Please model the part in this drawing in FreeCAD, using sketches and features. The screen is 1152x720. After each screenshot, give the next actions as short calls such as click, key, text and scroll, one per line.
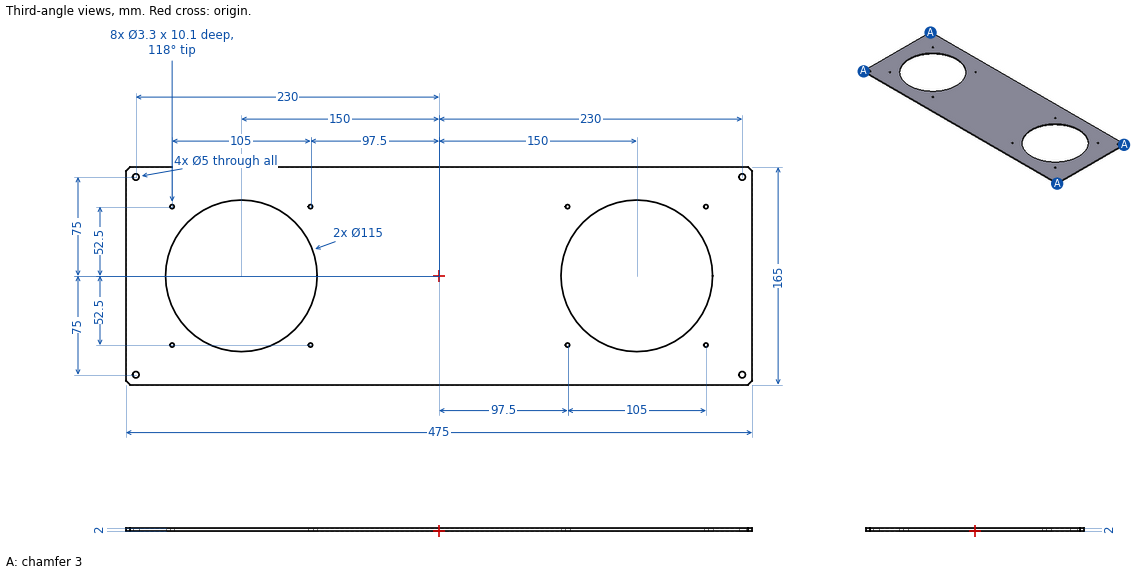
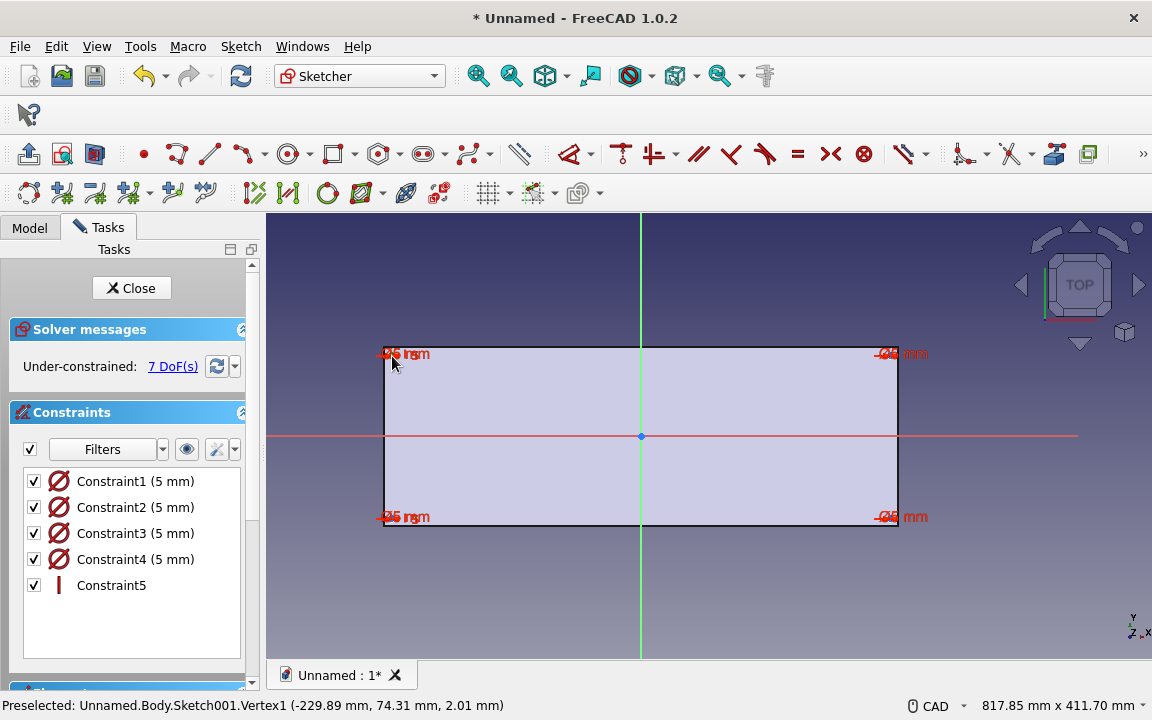
click(890, 356)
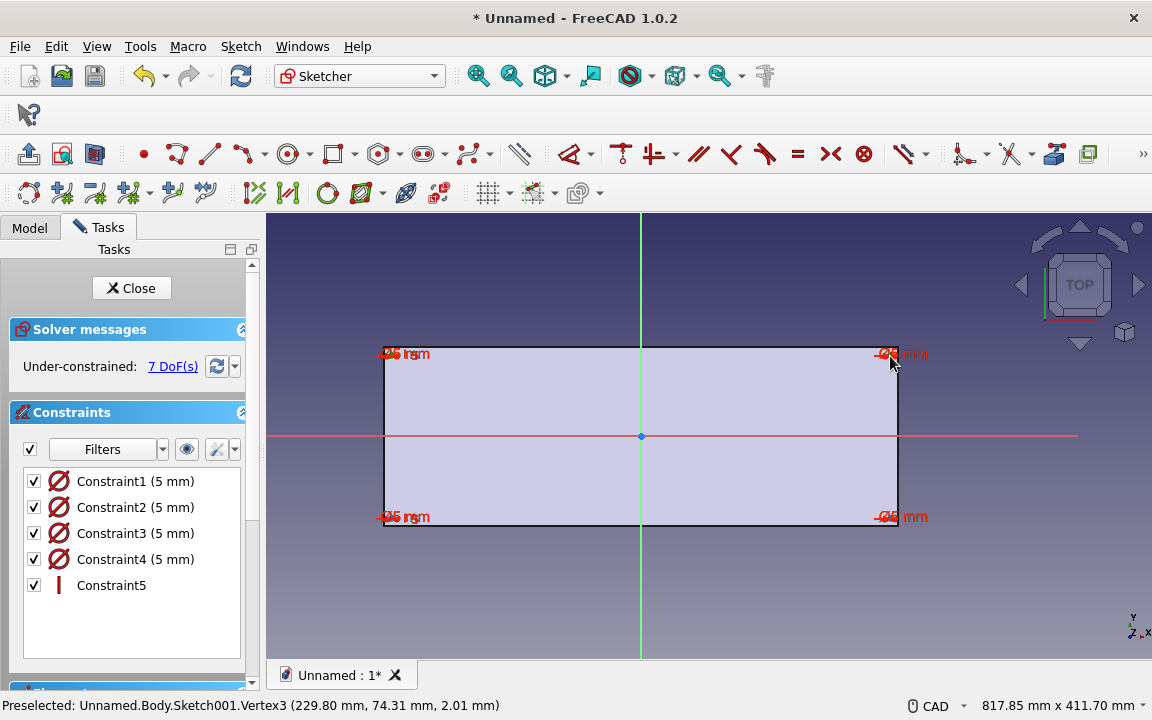
key(h)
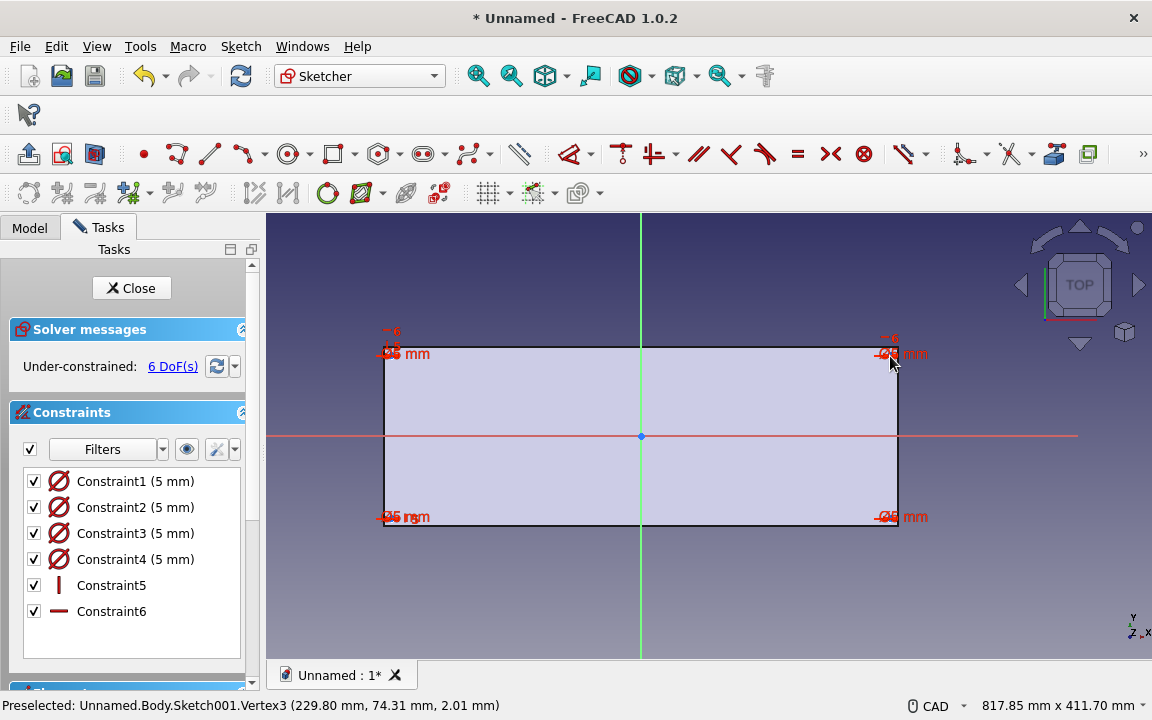
click(890, 356)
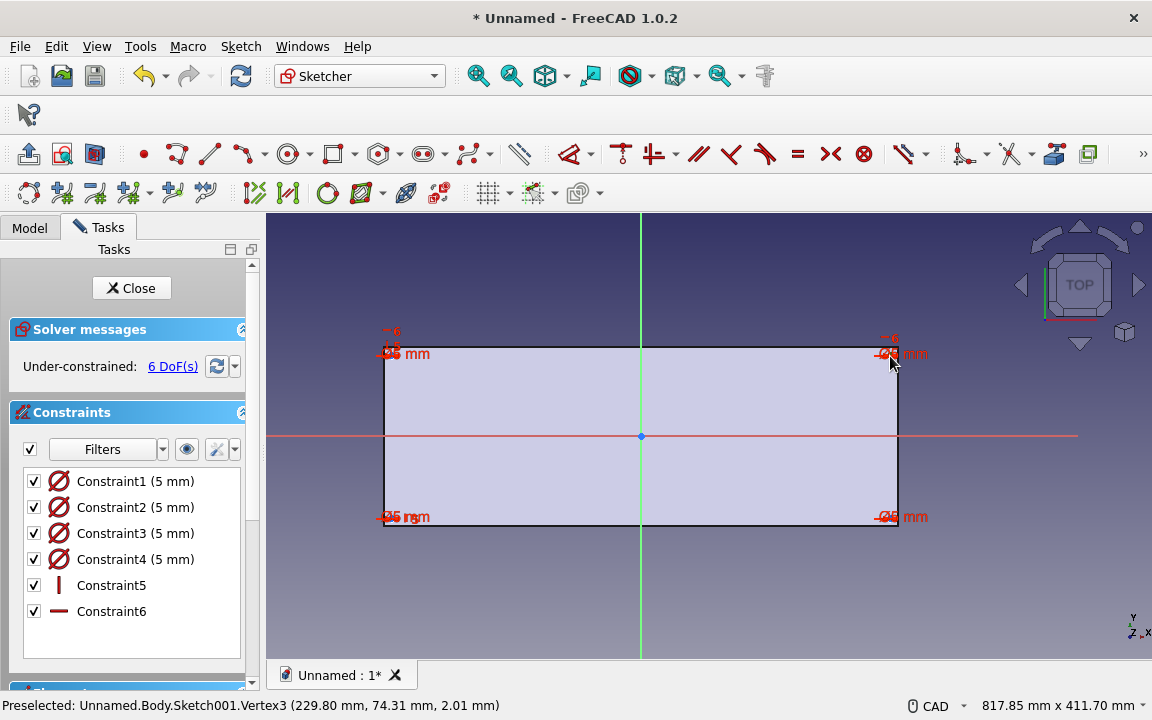
click(890, 519)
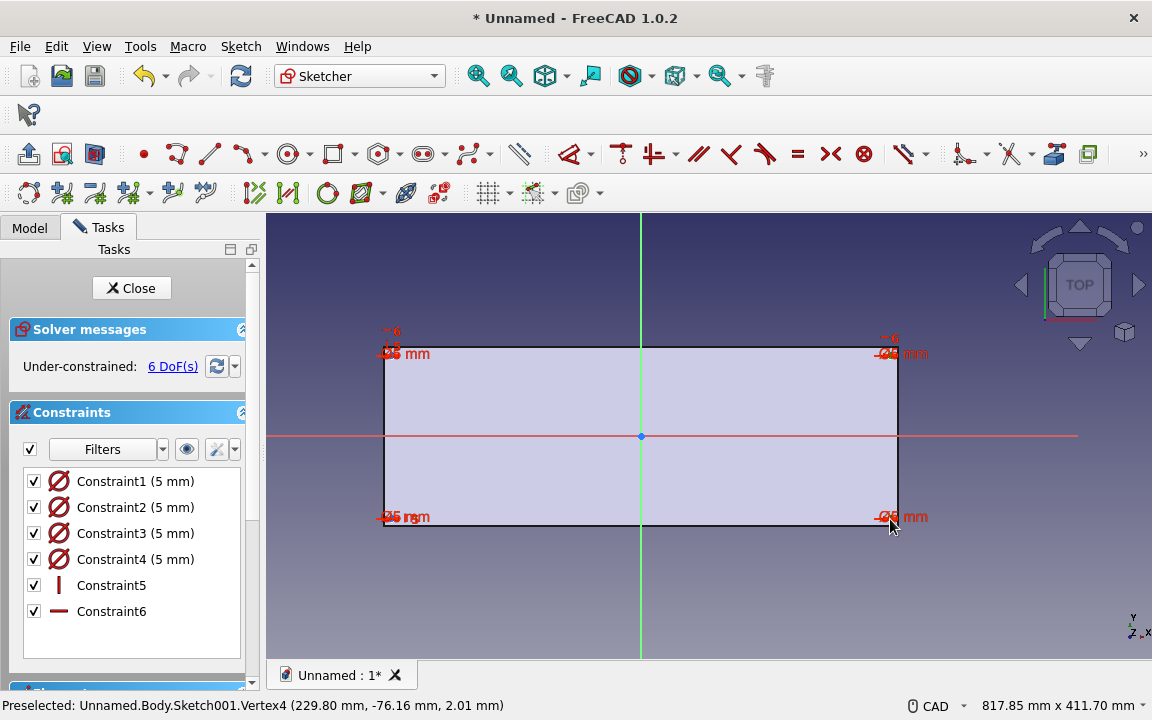
key(v)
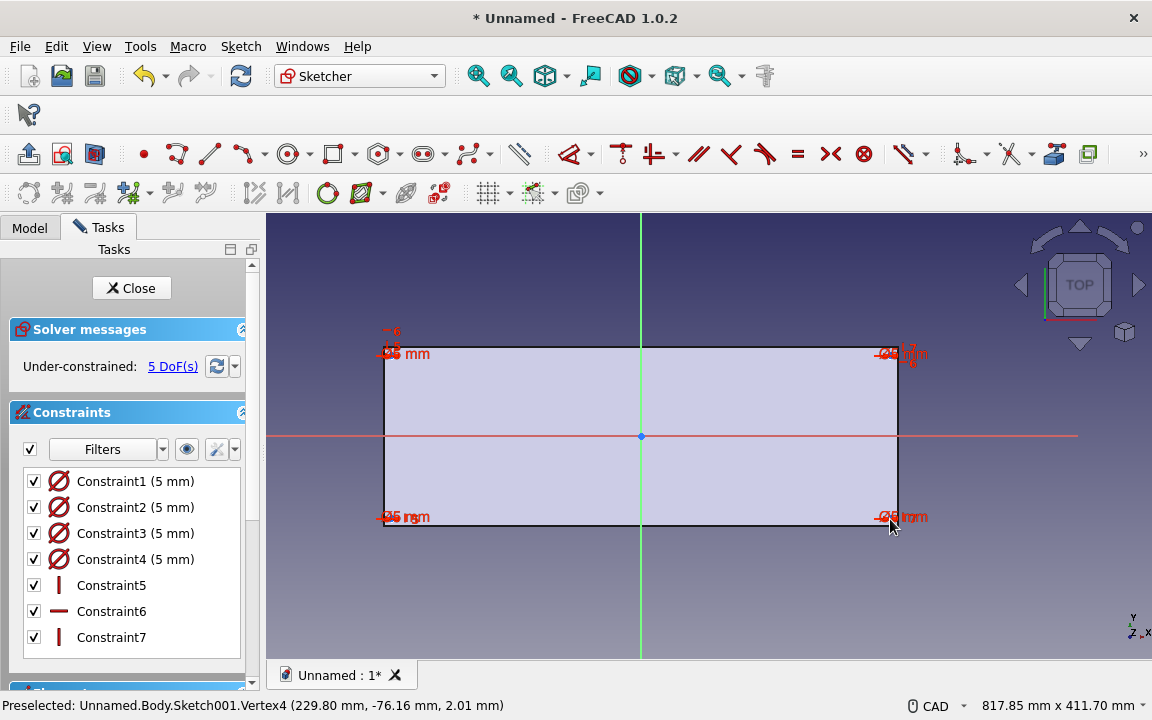
click(392, 519)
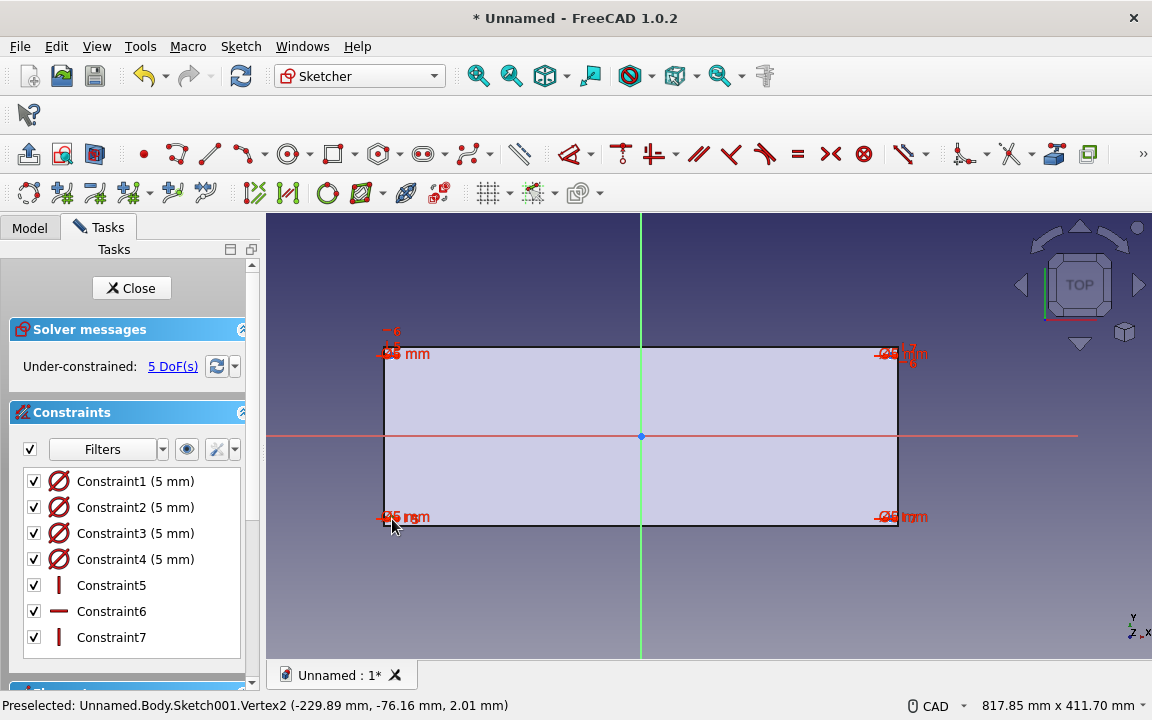
click(890, 519)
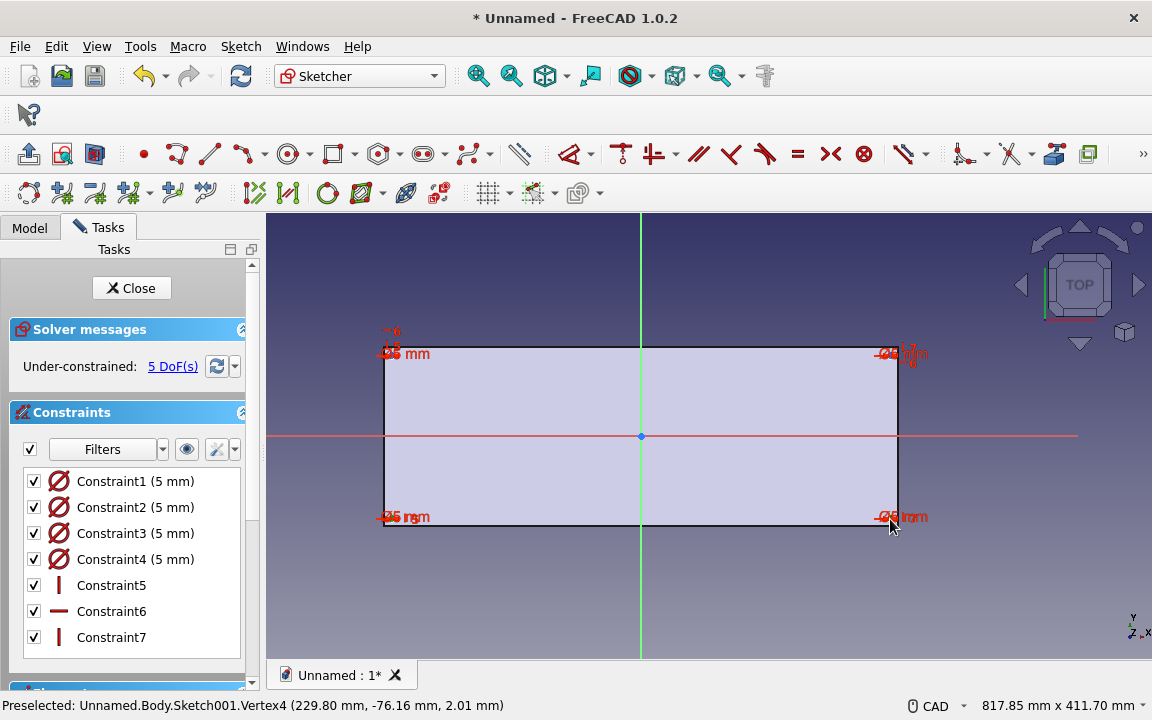
key(h)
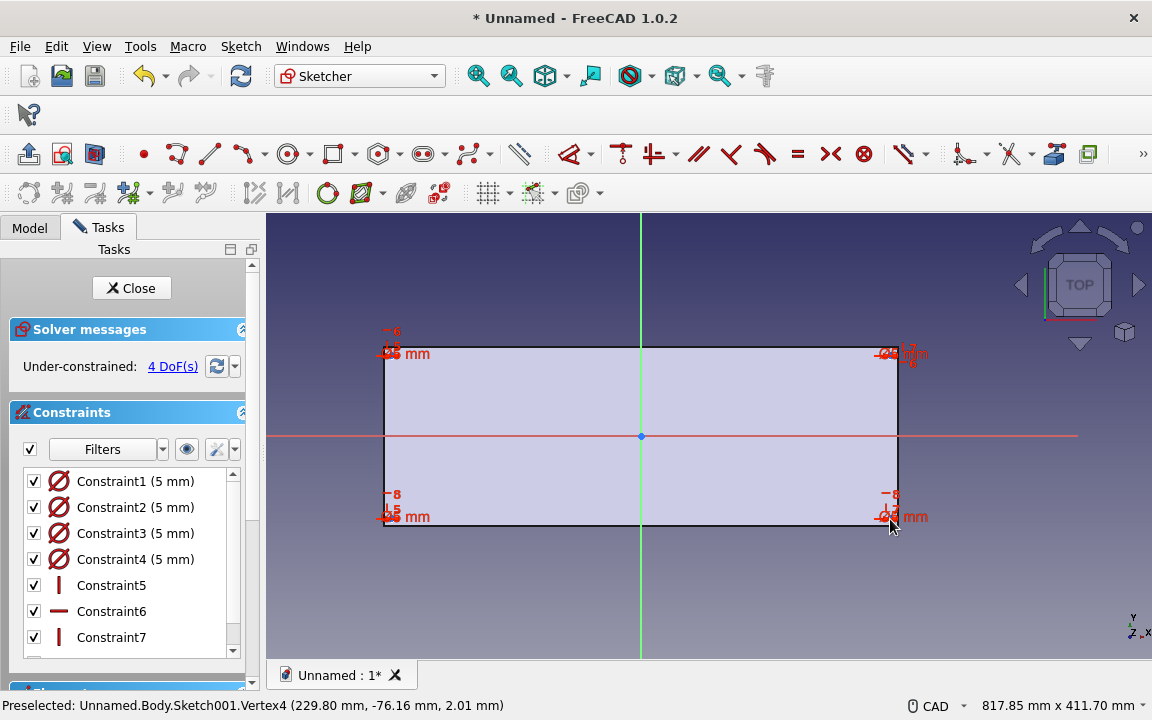
key(d)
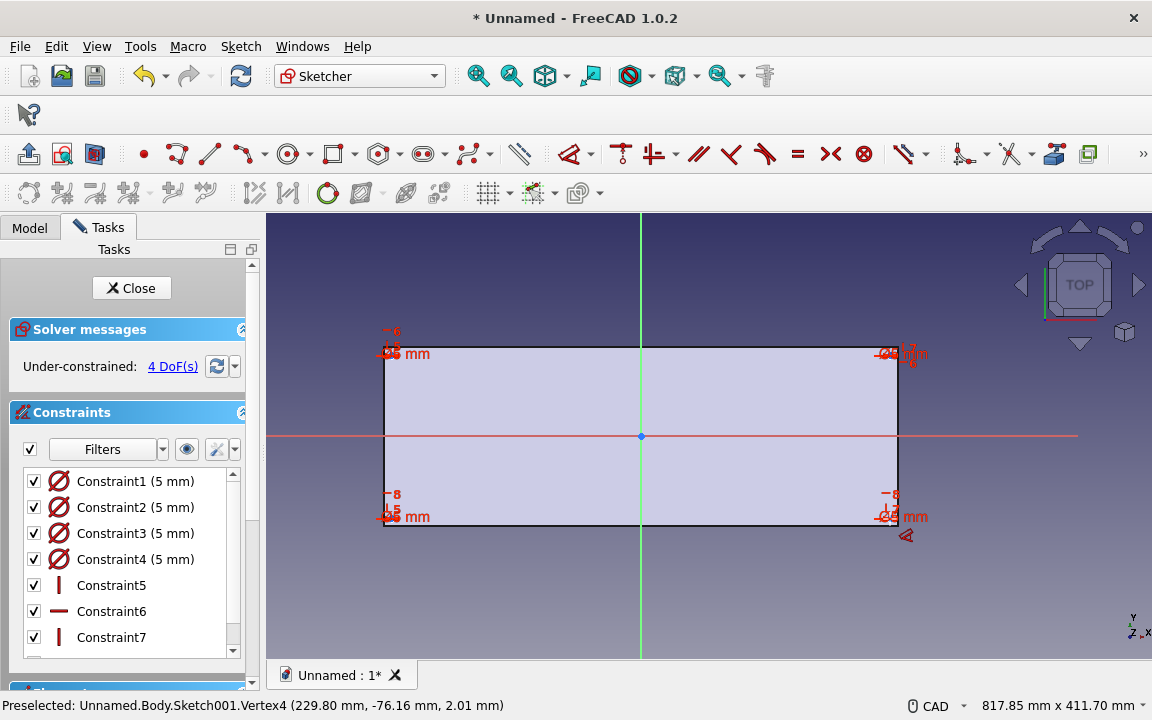
click(392, 356)
click(358, 396)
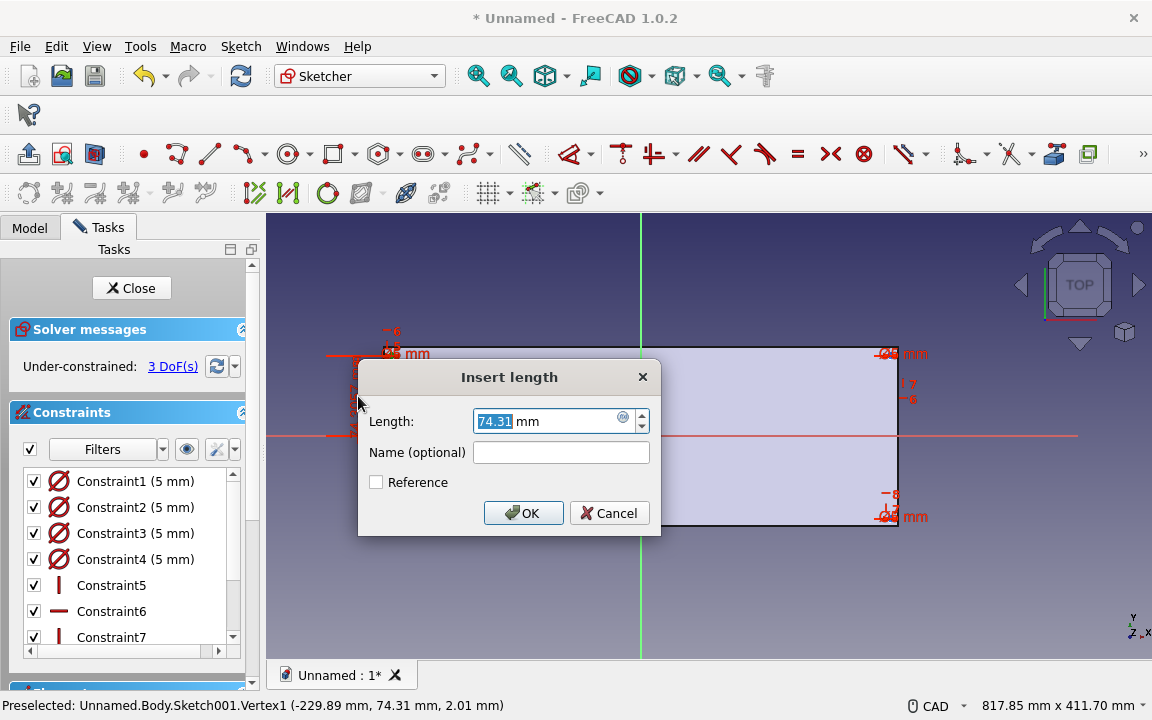
text(75)
key(Return)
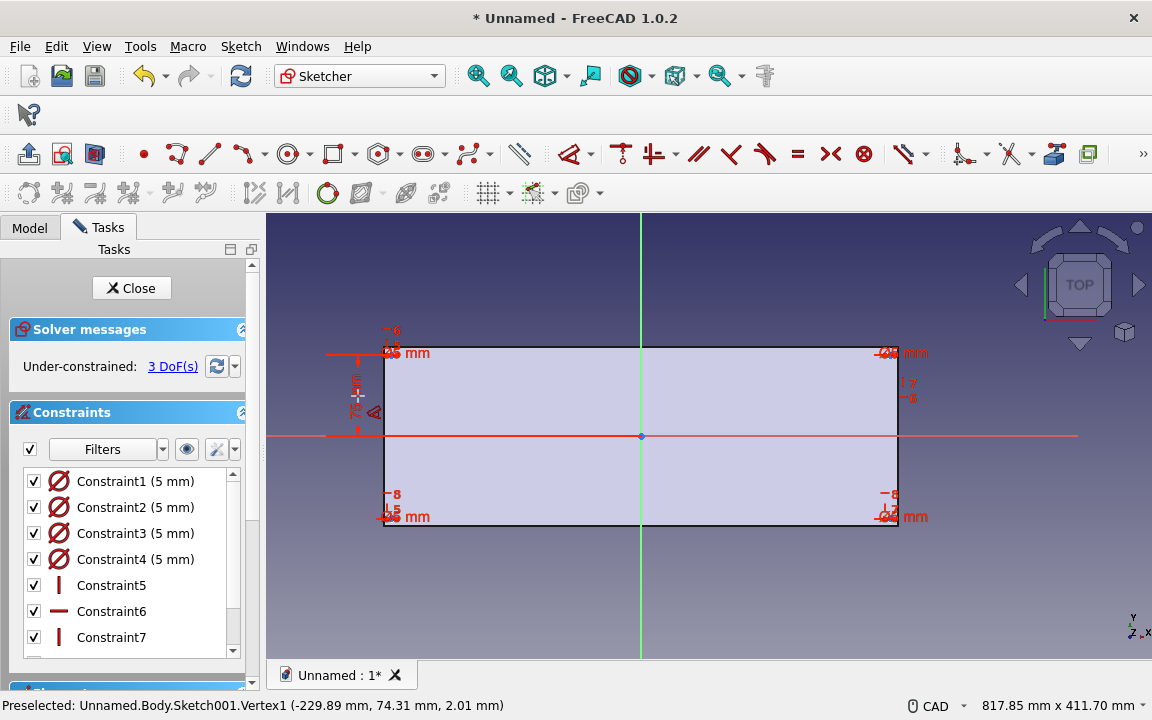
click(392, 519)
click(358, 478)